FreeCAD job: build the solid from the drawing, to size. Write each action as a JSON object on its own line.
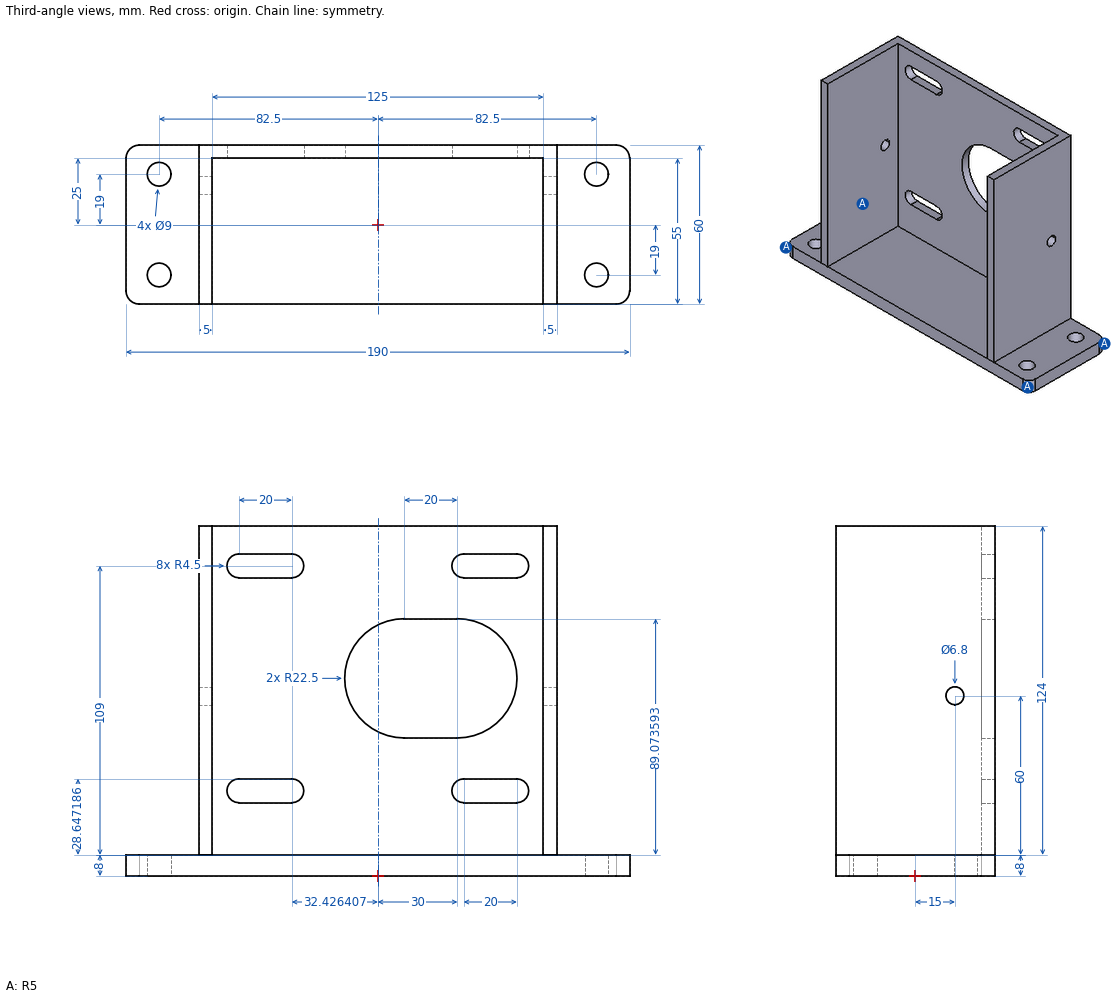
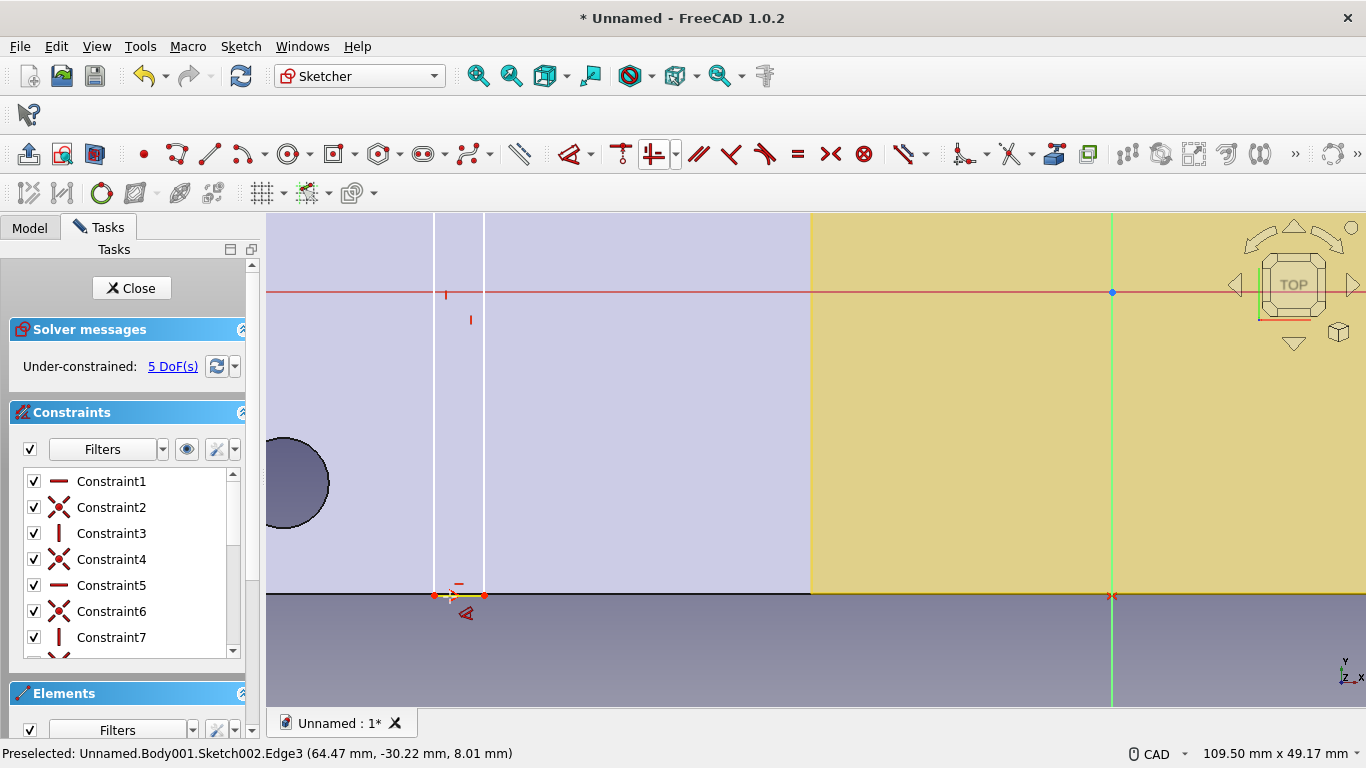
{"action": "left_click", "coordinate": [449, 596]}
{"action": "left_click", "coordinate": [459, 630]}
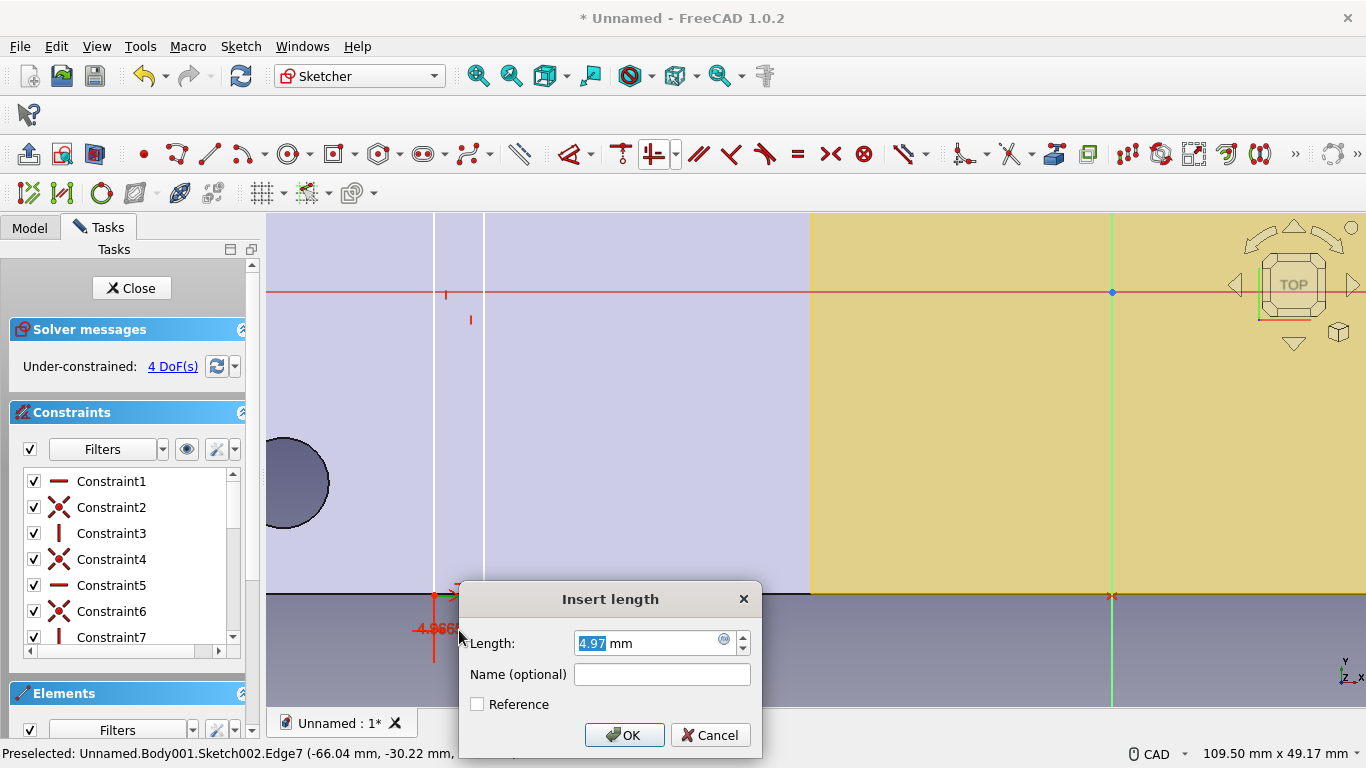
{"action": "type", "text": "5"}
{"action": "key", "text": "Return"}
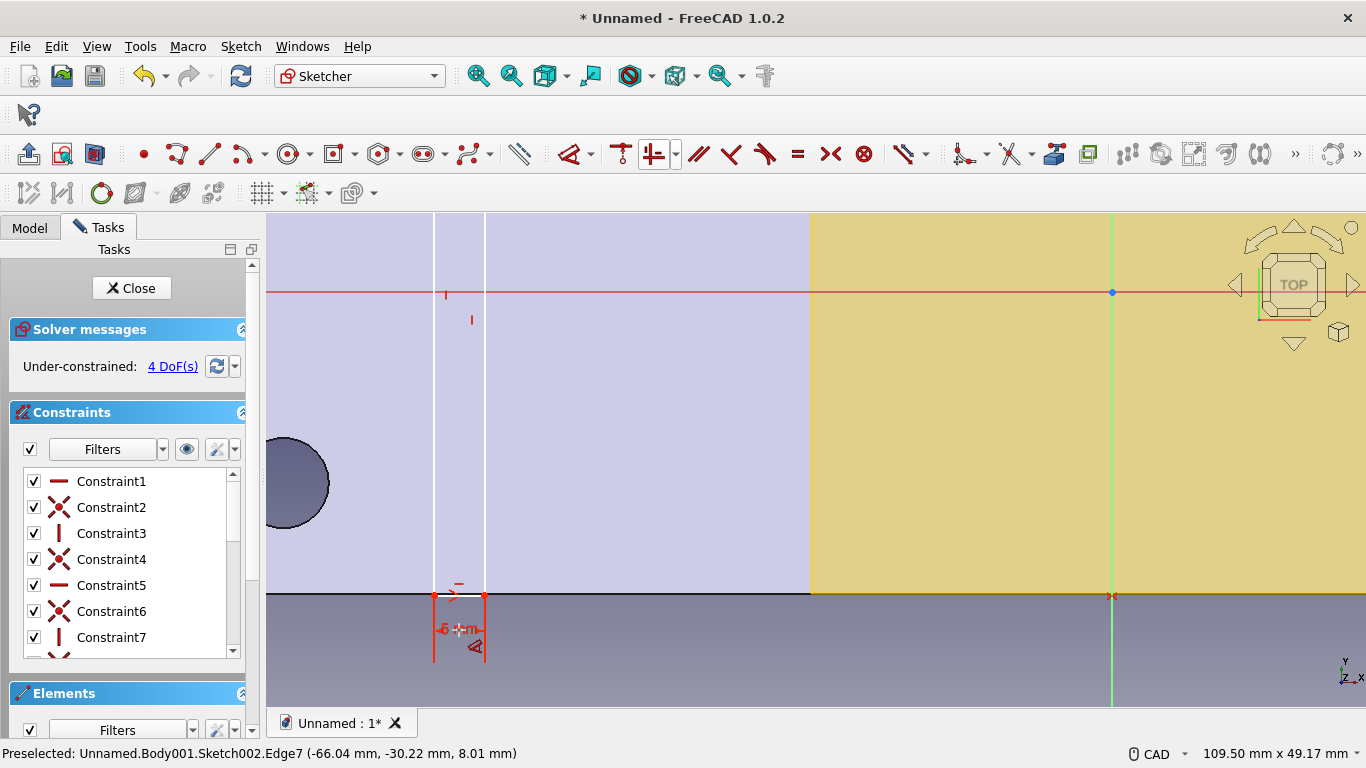
{"action": "scroll", "coordinate": [450, 597], "scroll_direction": "down", "scroll_amount": 4}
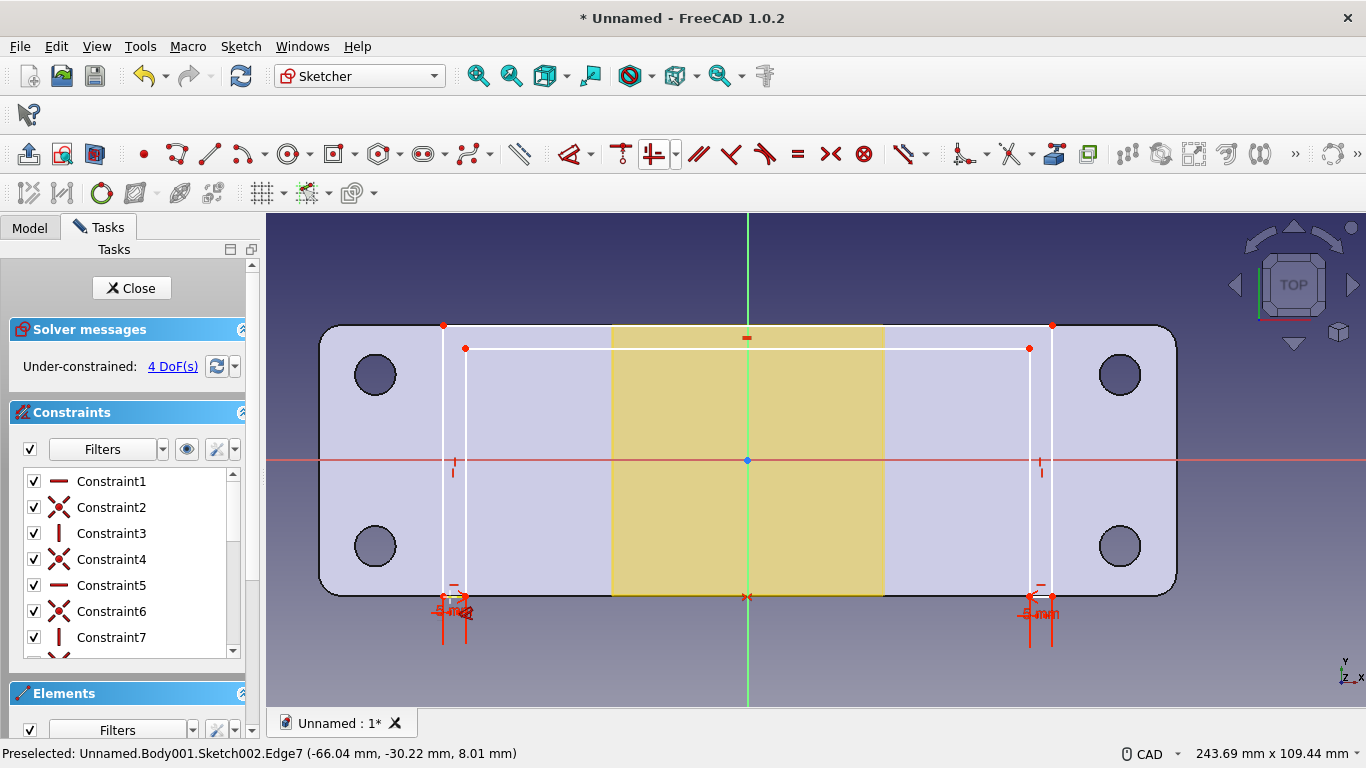
{"action": "left_click", "coordinate": [1030, 423]}
{"action": "left_click", "coordinate": [996, 416]}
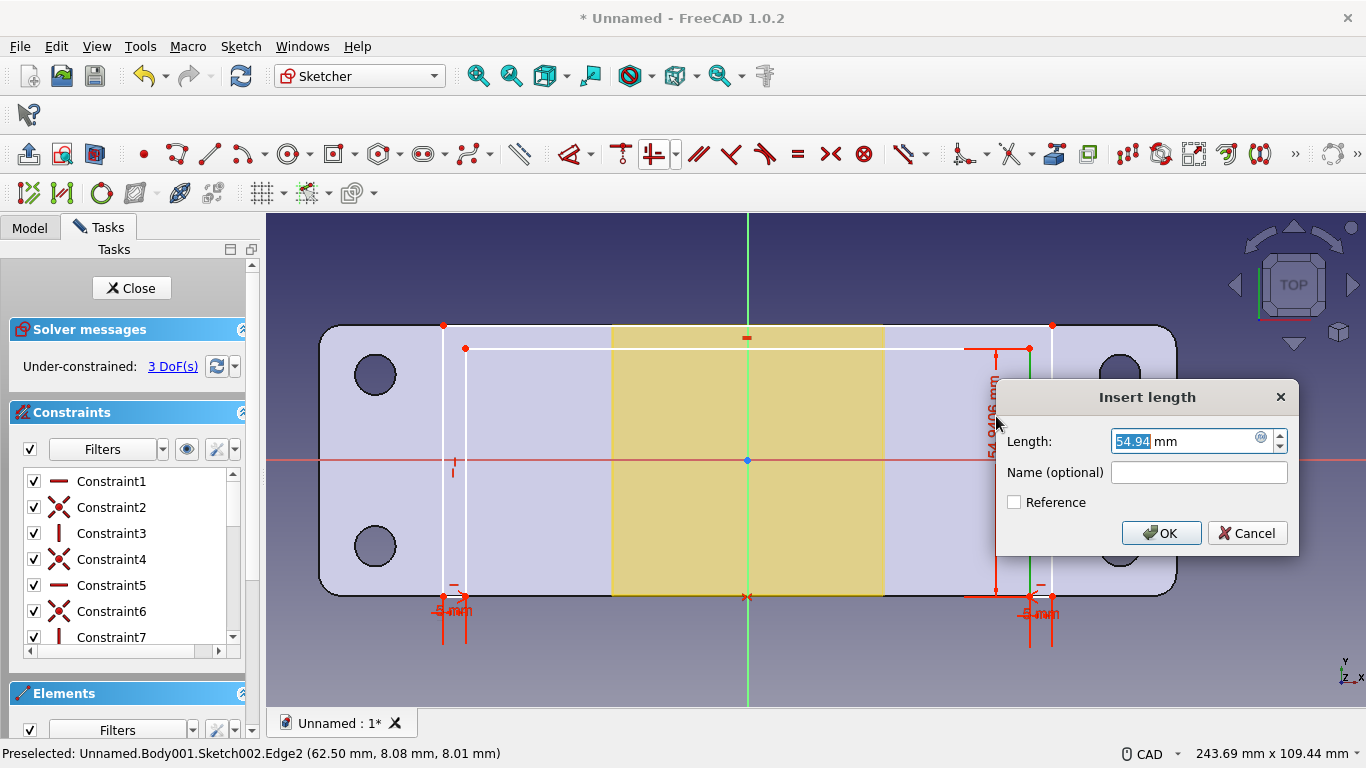
{"action": "type", "text": "55"}
{"action": "key", "text": "Return"}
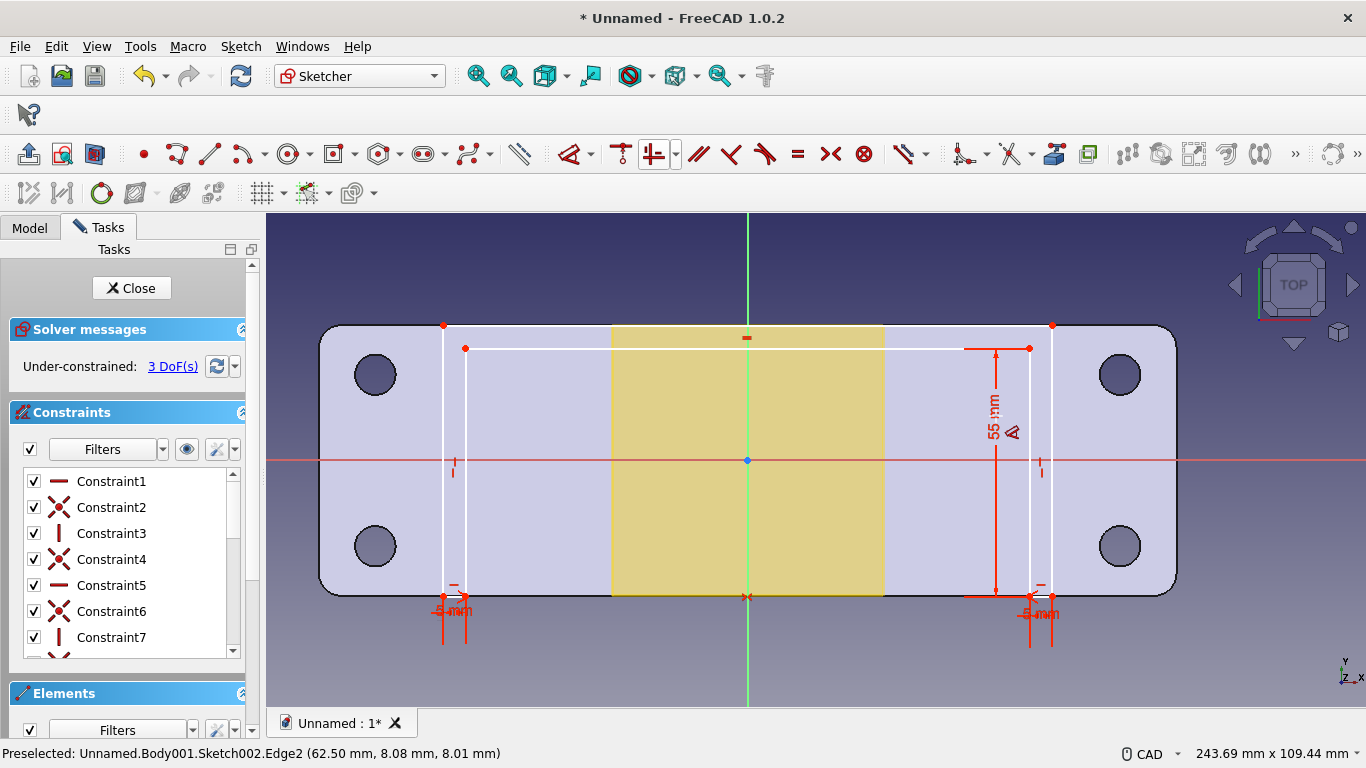
{"action": "left_click", "coordinate": [1052, 516]}
{"action": "left_click", "coordinate": [1086, 399]}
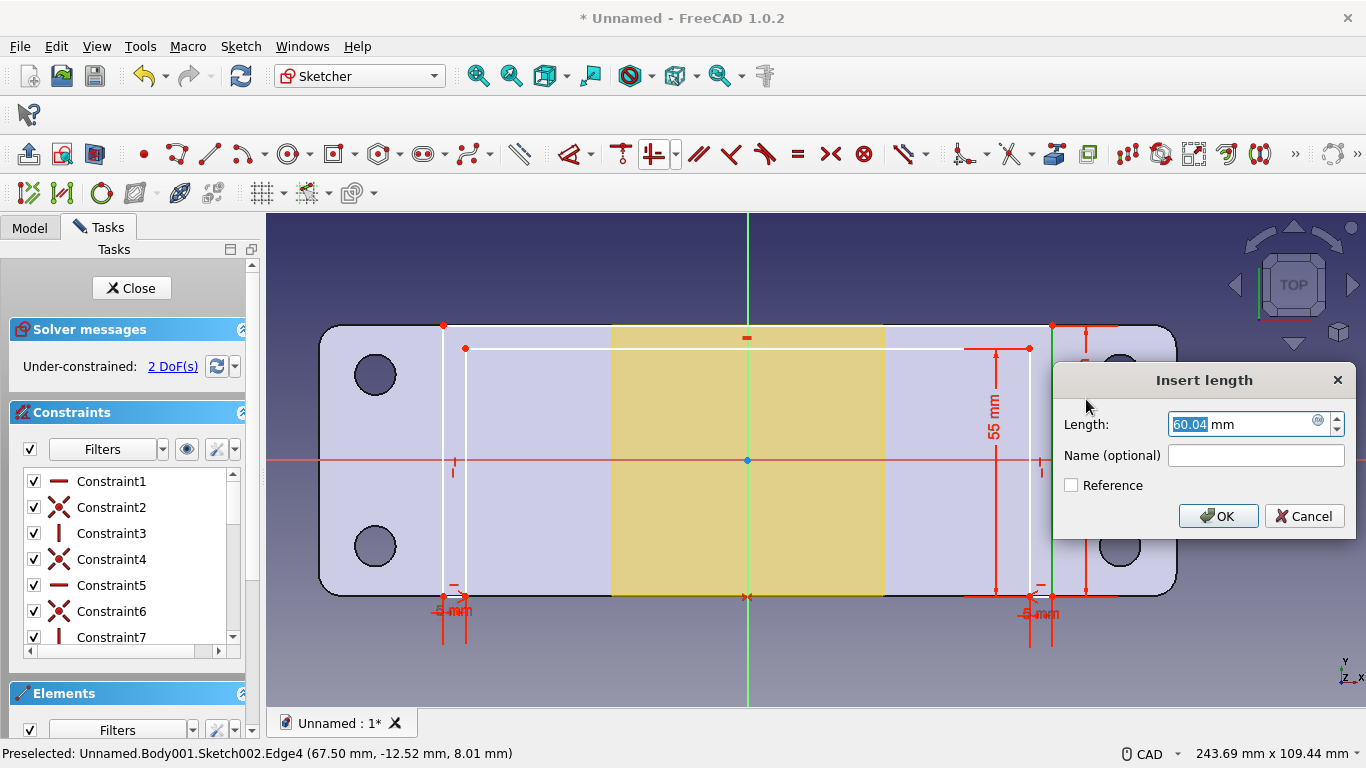
{"action": "type", "text": "60"}
{"action": "key", "text": "Return"}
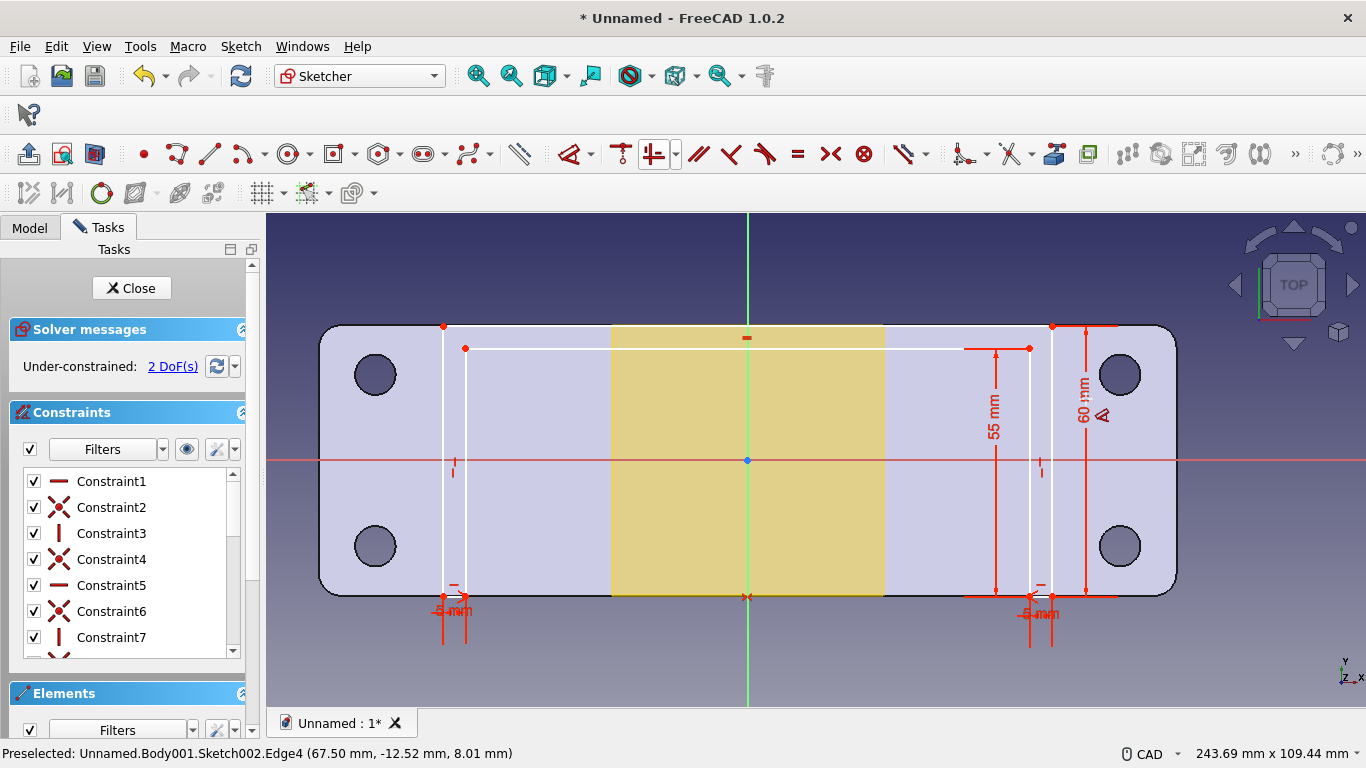
{"action": "left_click", "coordinate": [635, 349]}
{"action": "left_click", "coordinate": [618, 383]}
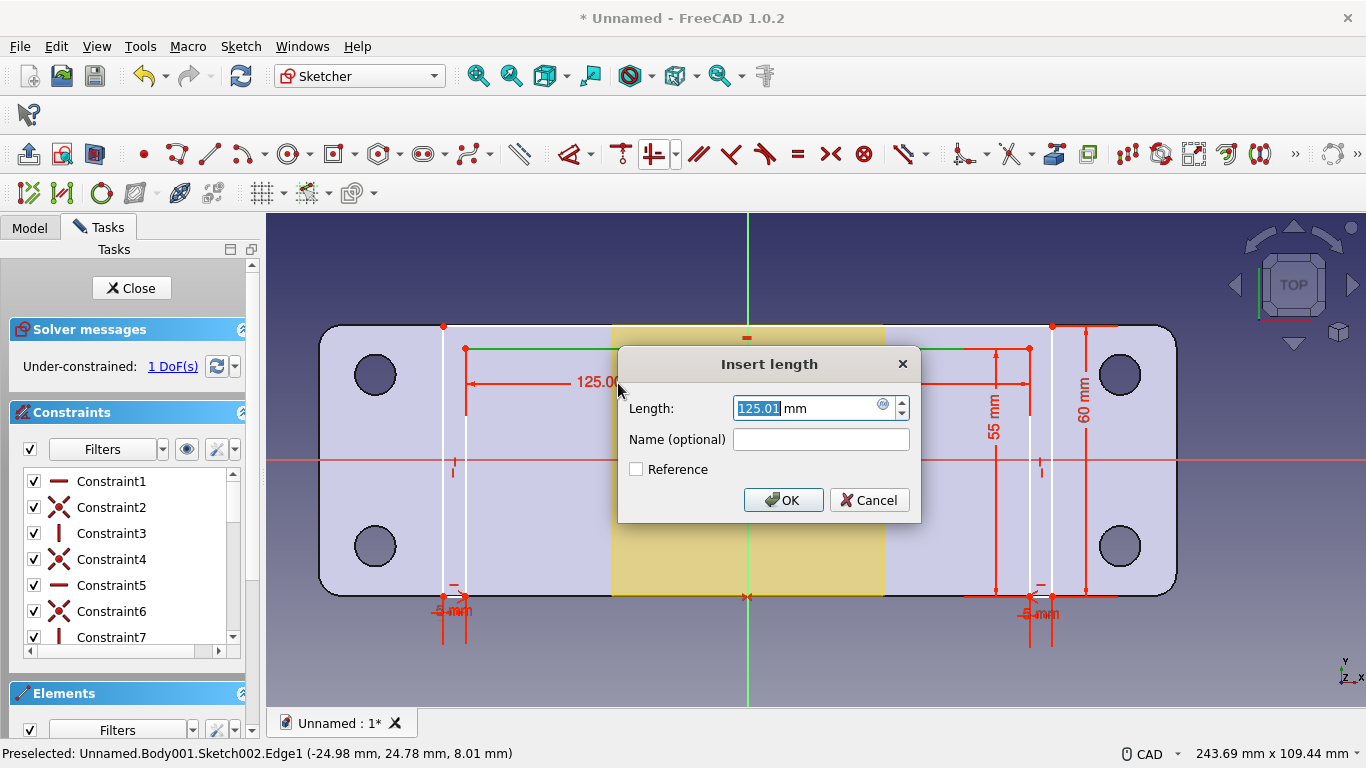
{"action": "type", "text": "125"}
{"action": "key", "text": "Return"}